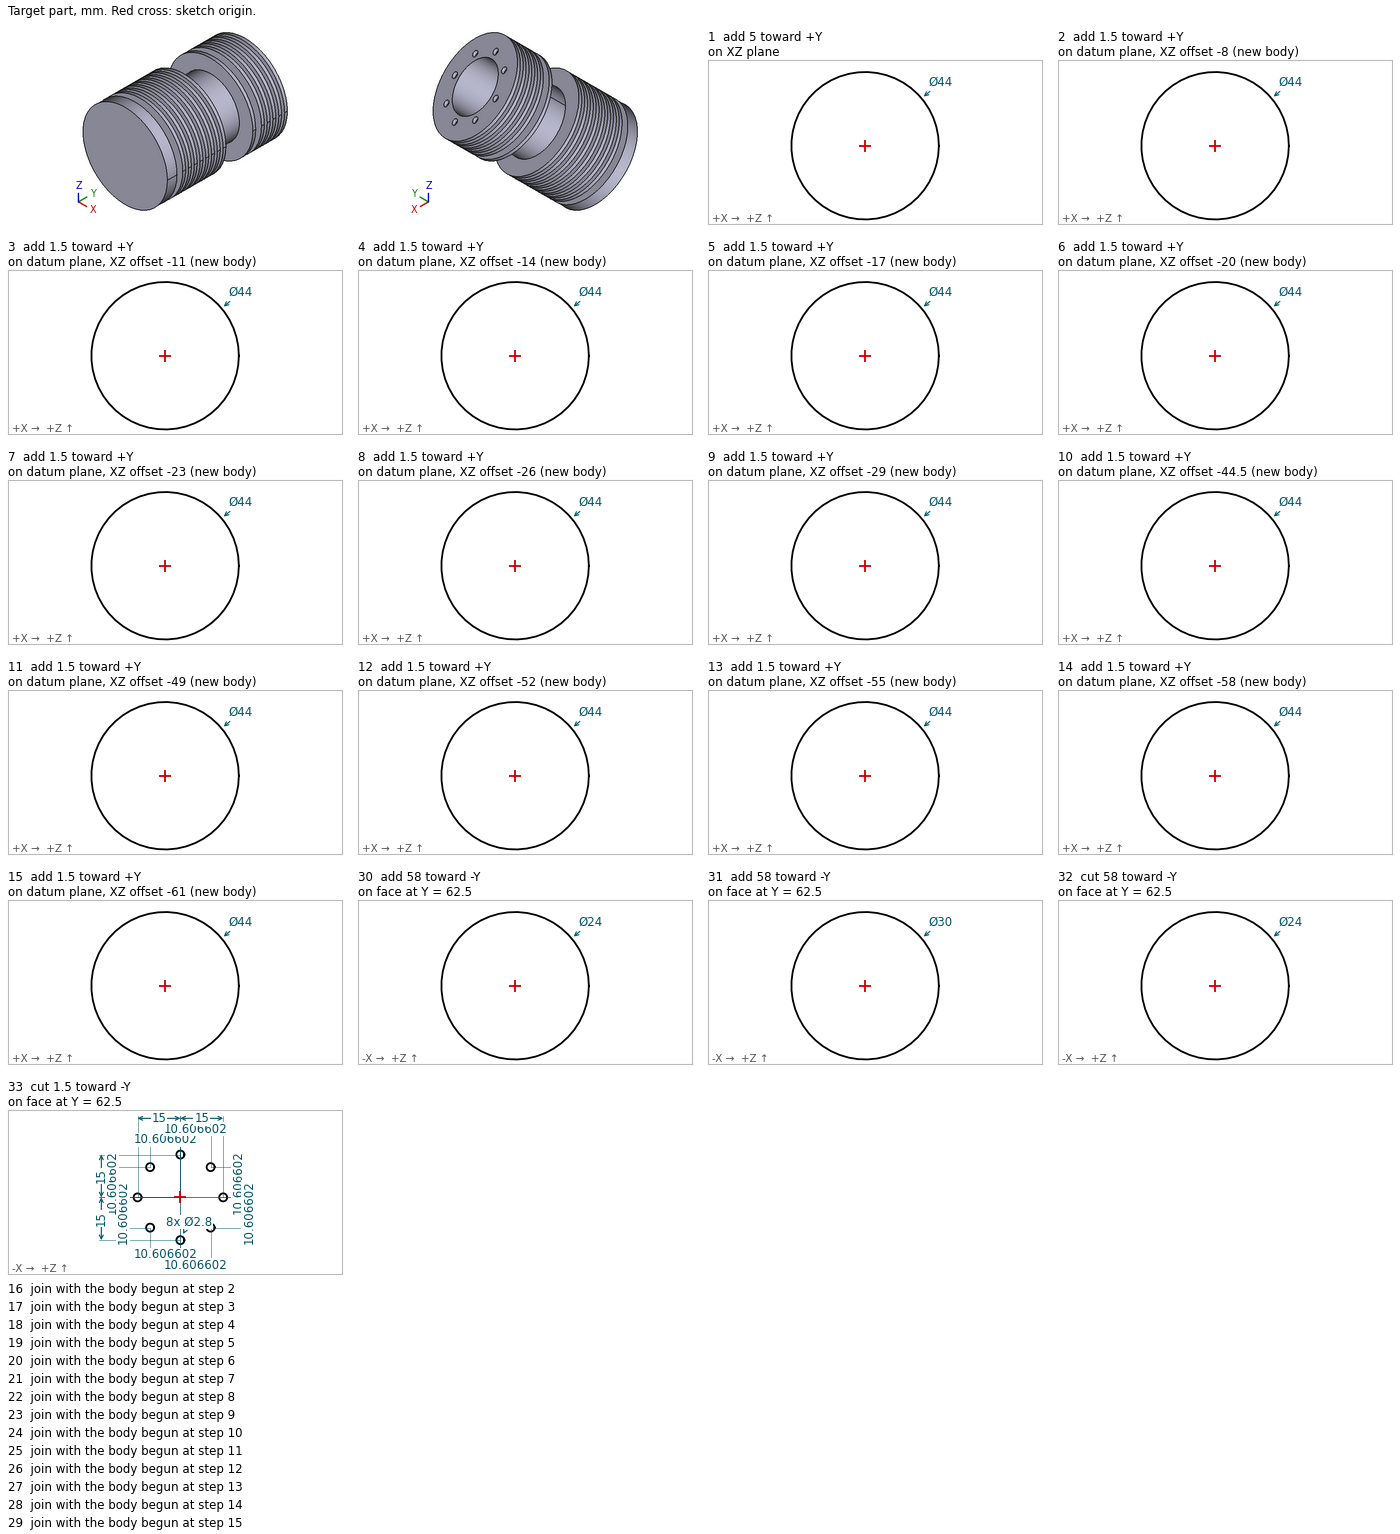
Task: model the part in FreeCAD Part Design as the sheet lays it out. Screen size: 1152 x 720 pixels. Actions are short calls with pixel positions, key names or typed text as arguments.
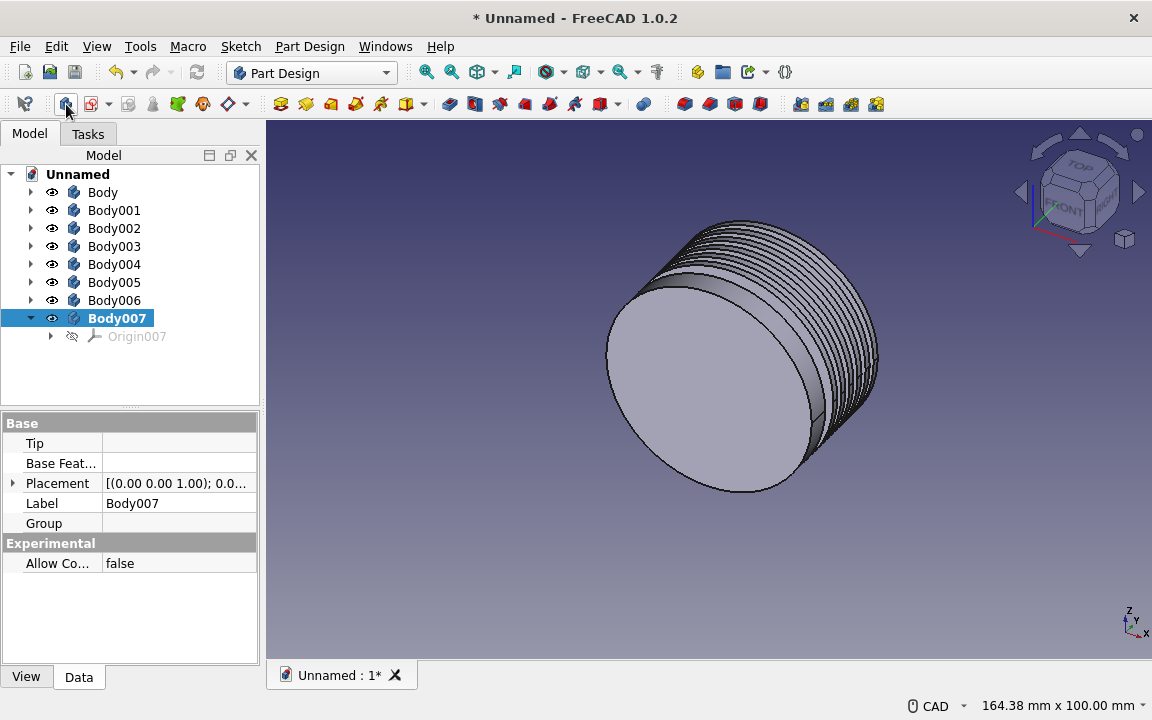
click(51, 336)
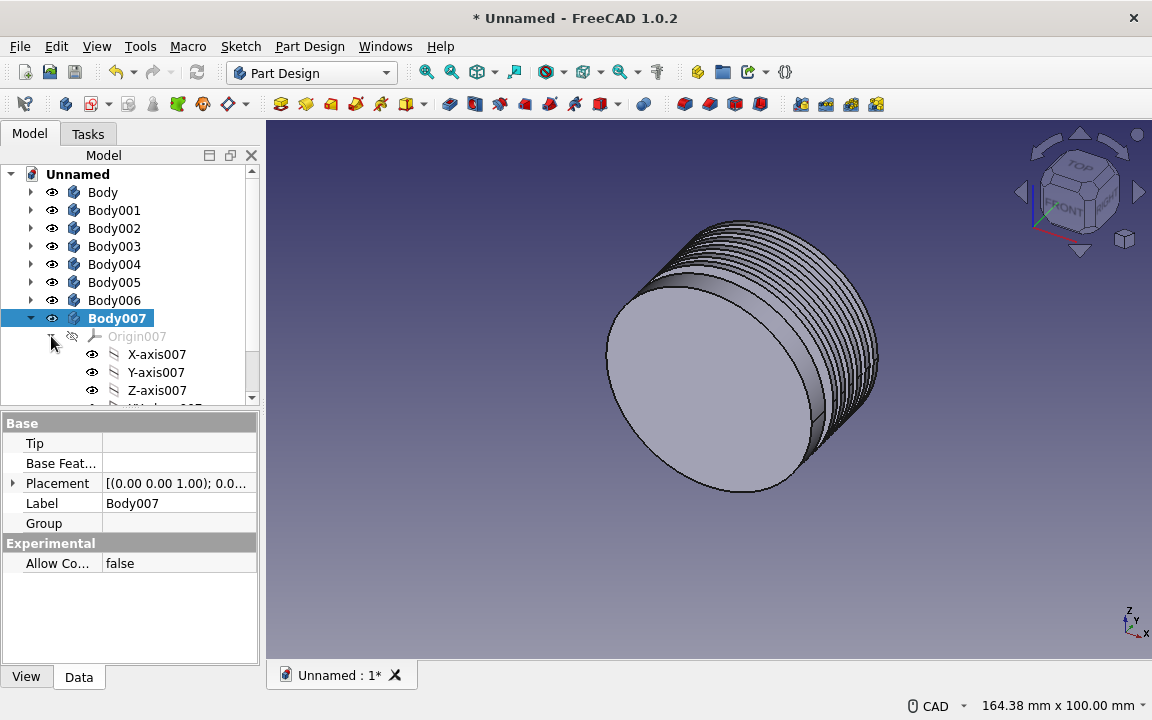
scroll(101, 278, down, 3)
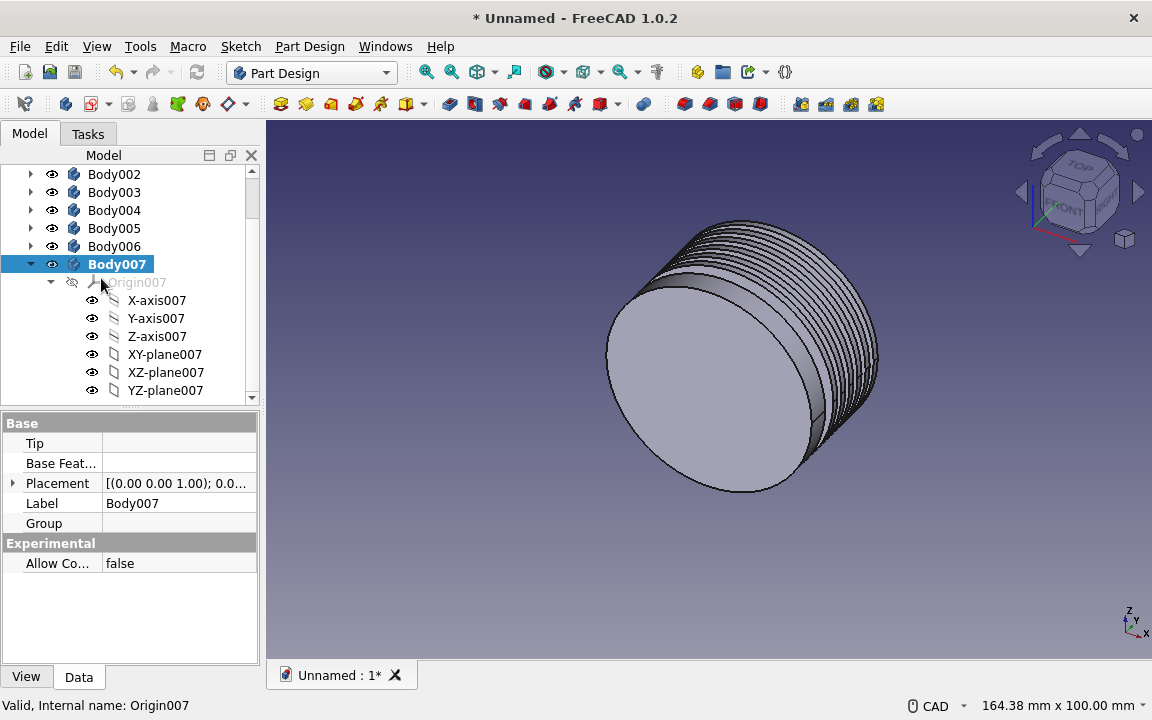
click(137, 372)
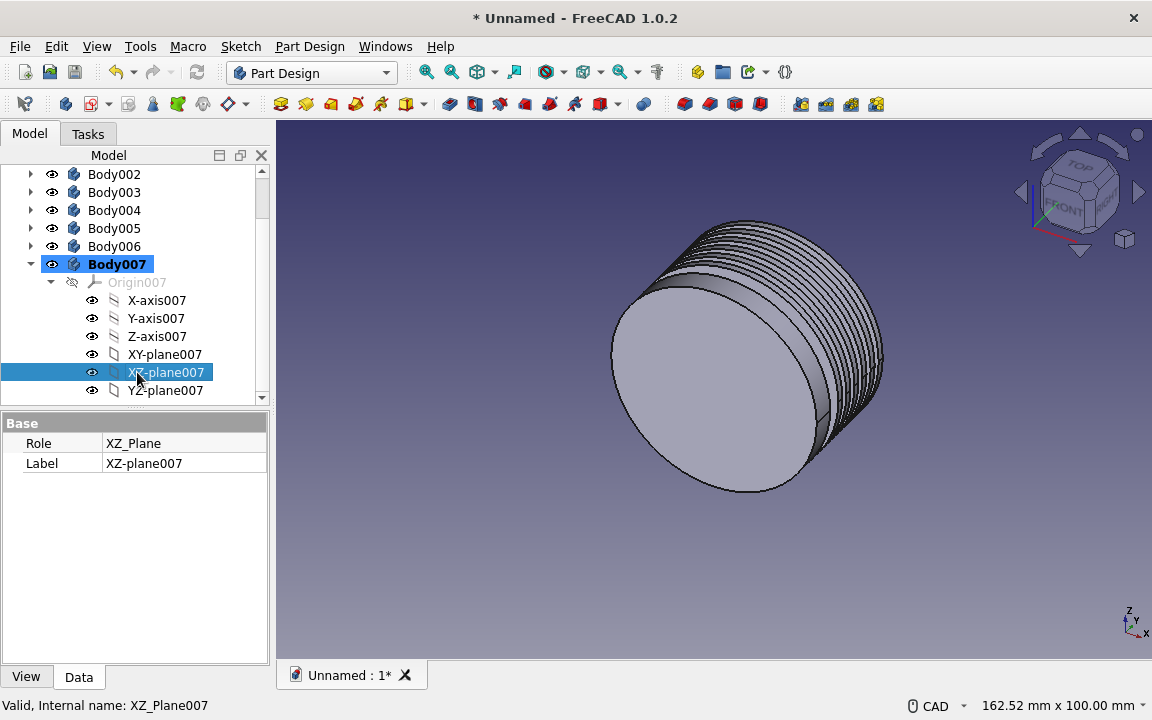
click(228, 104)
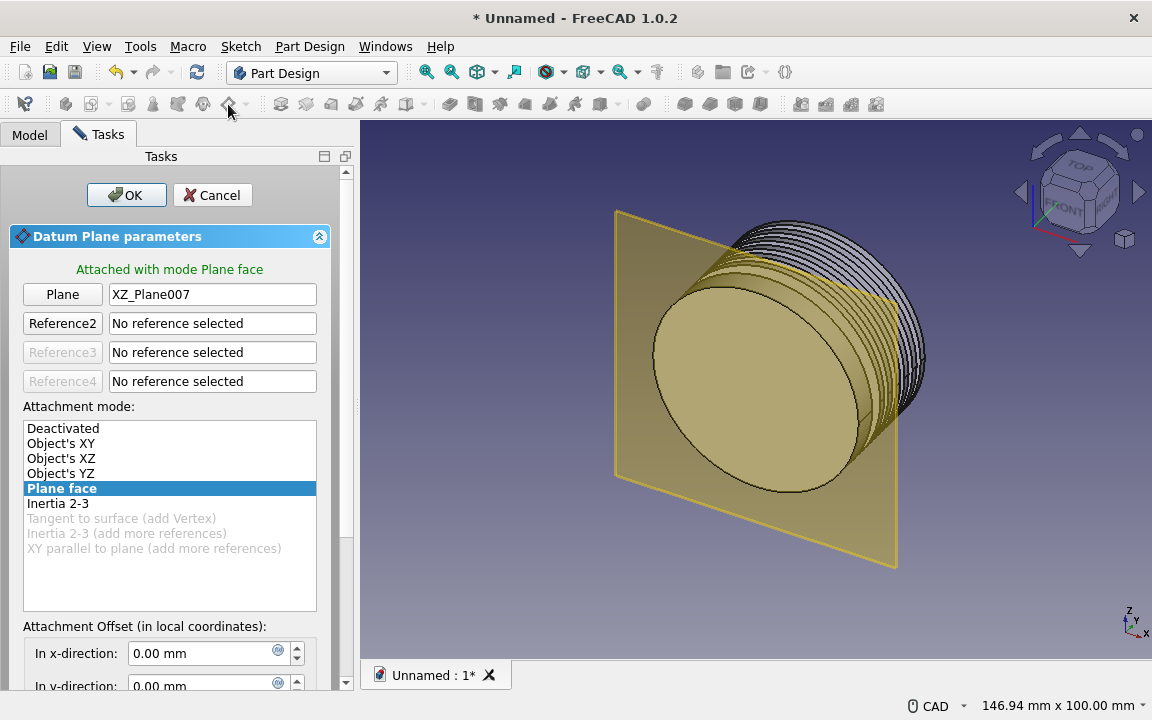
scroll(346, 428, down, 2)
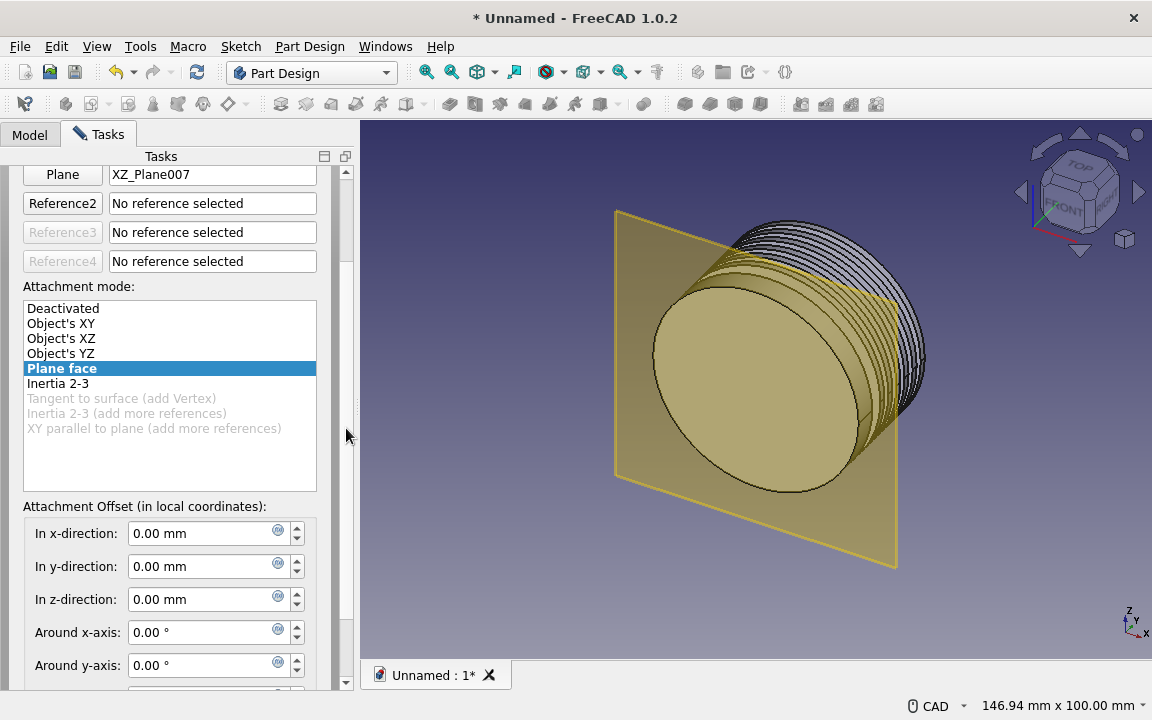
triple_click(210, 600)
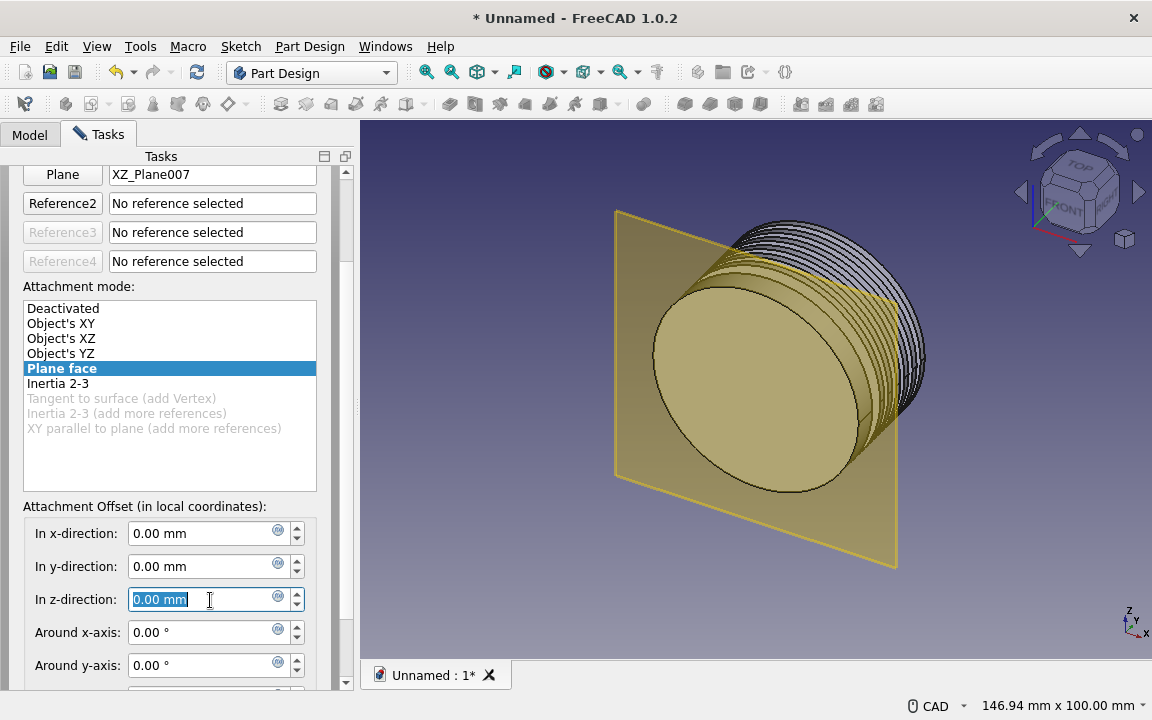
text(-26)
key(Tab)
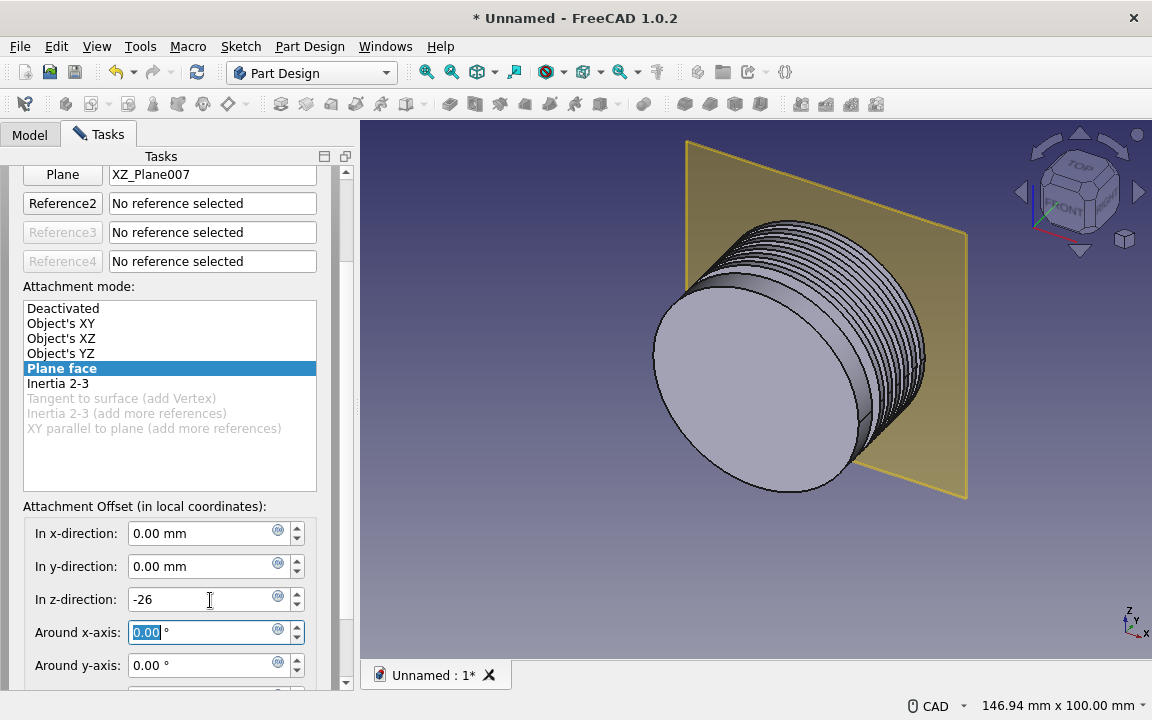
scroll(346, 428, up, 3)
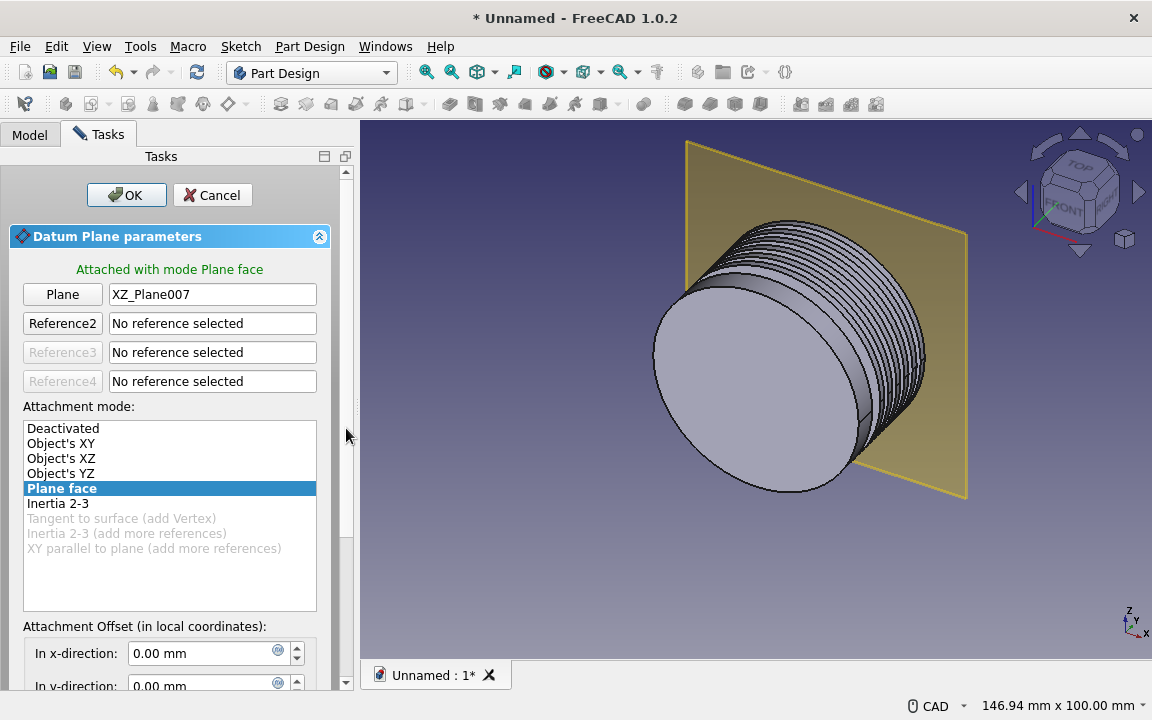
click(127, 195)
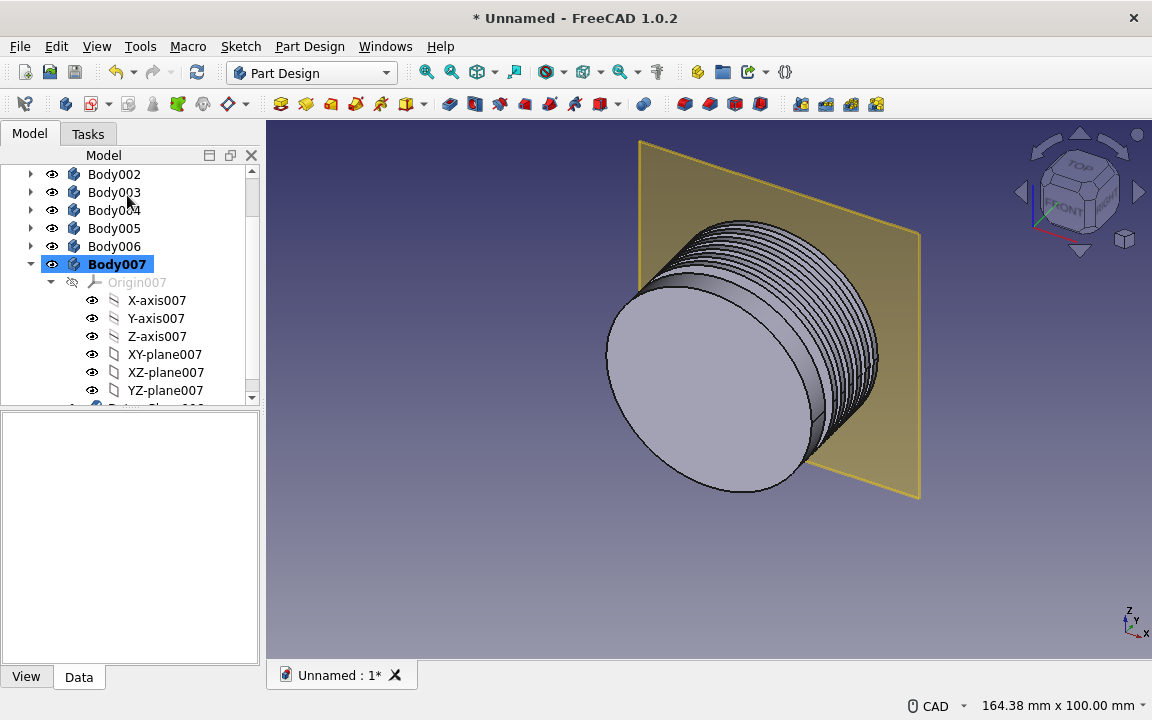
scroll(121, 278, down, 3)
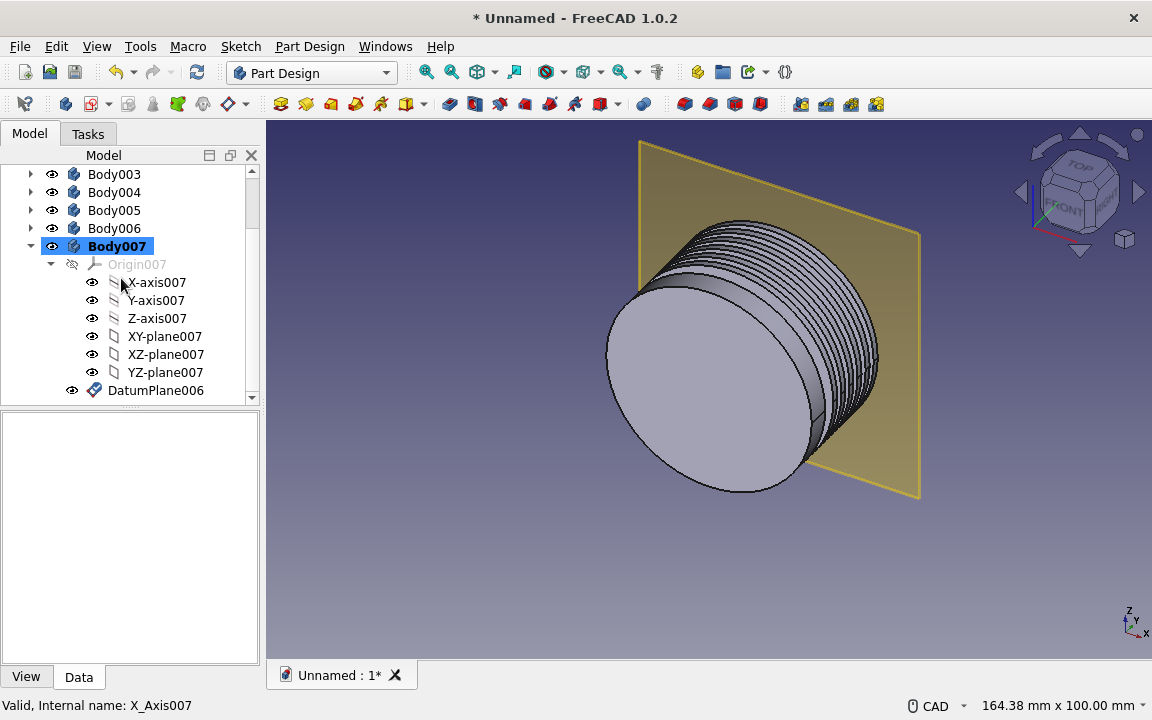
click(117, 390)